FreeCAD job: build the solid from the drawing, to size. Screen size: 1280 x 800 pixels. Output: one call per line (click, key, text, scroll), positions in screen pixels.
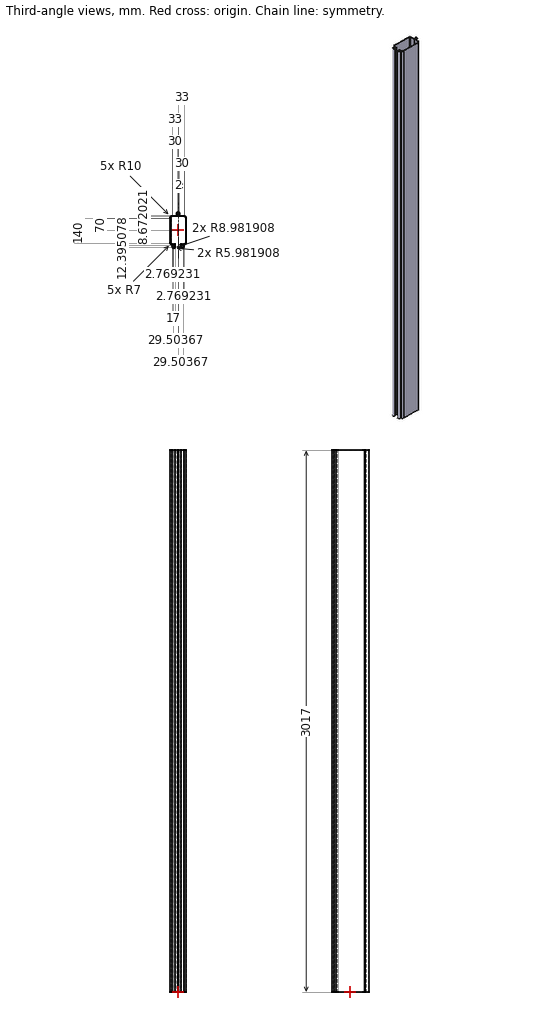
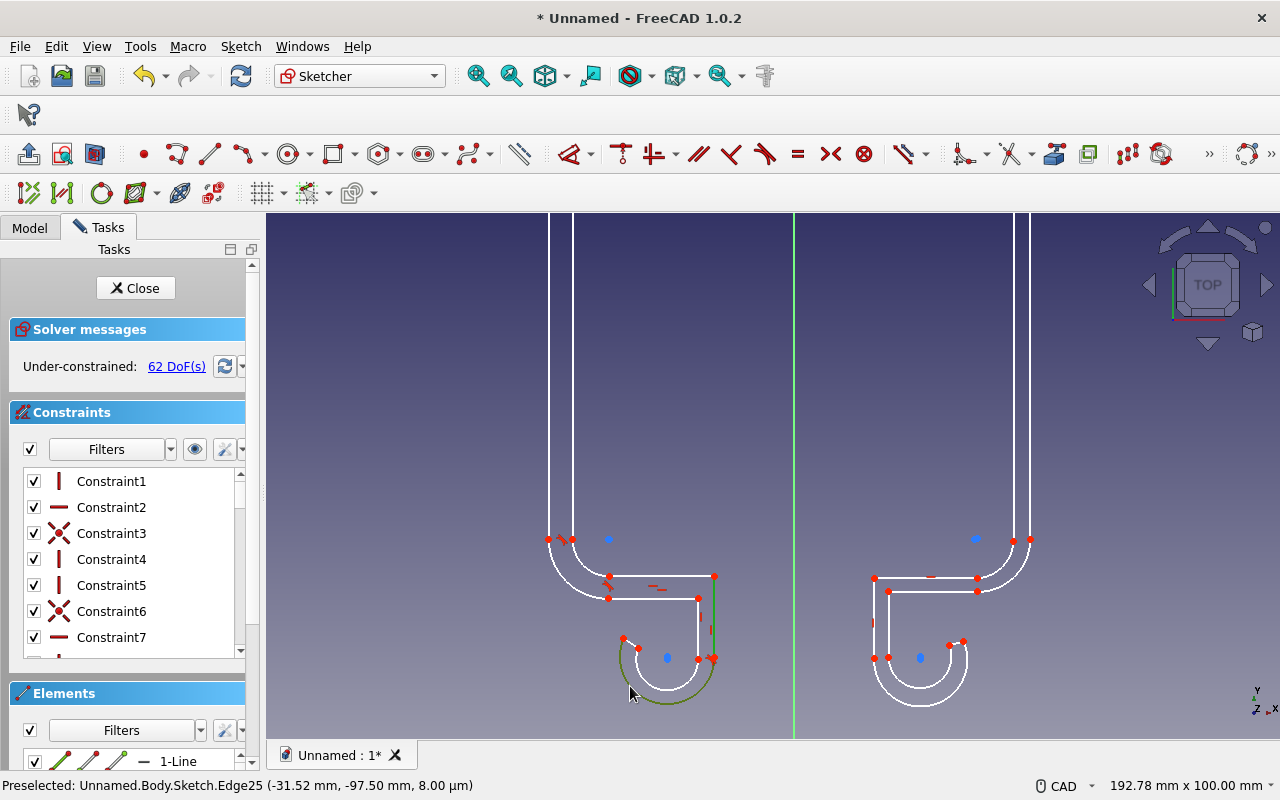
click(765, 154)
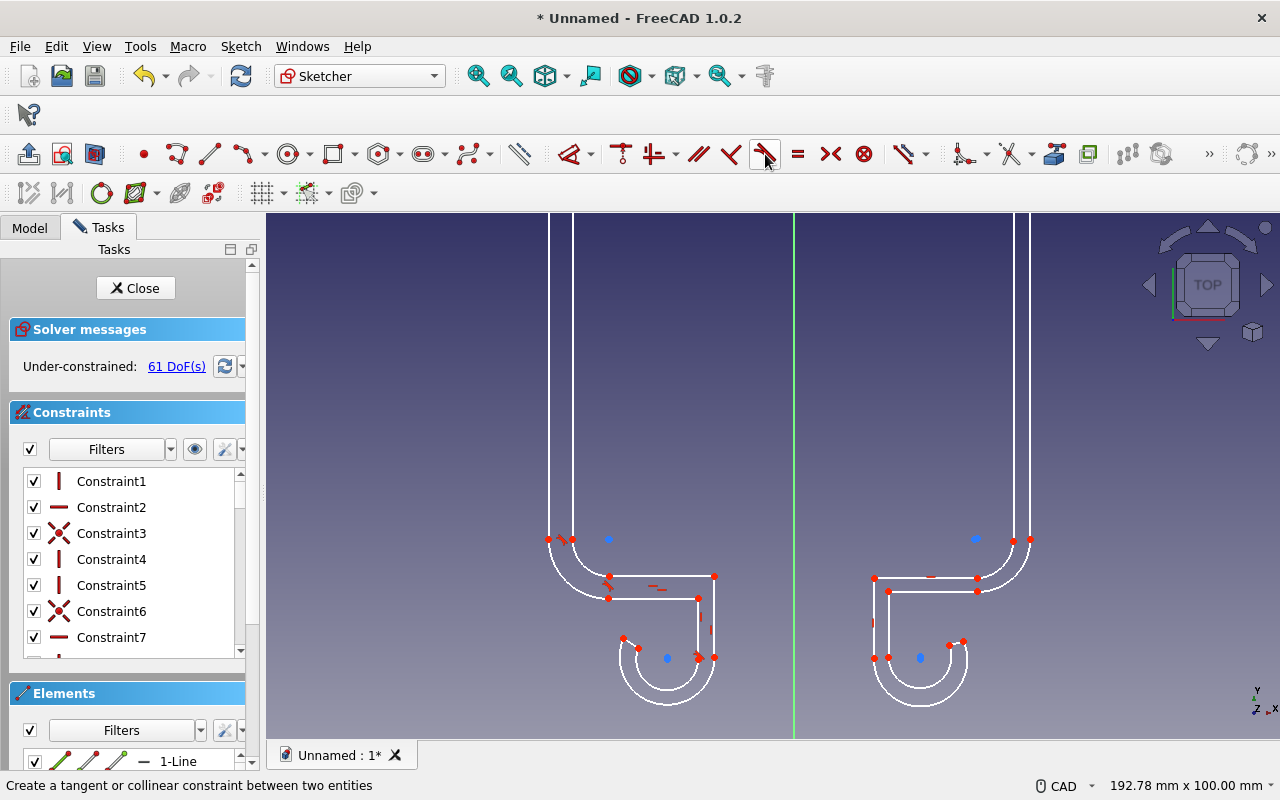
click(683, 576)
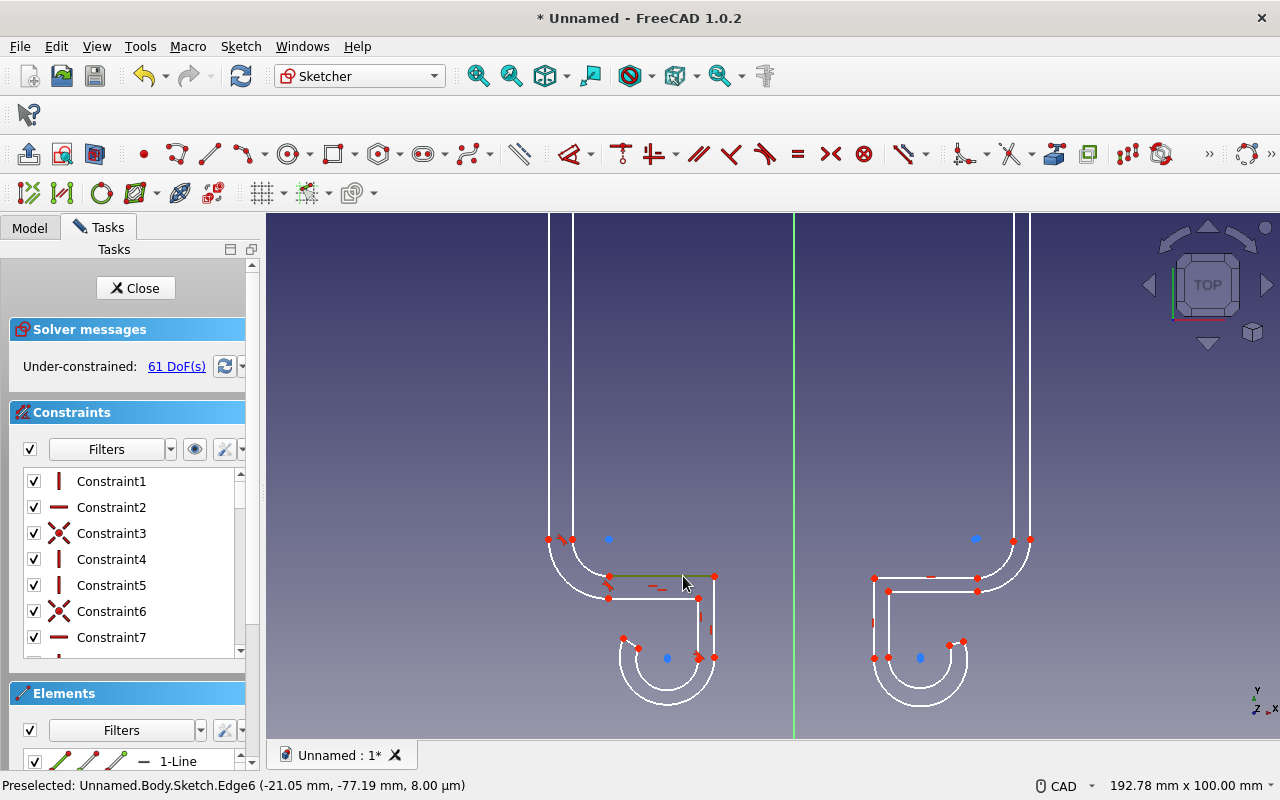
click(577, 556)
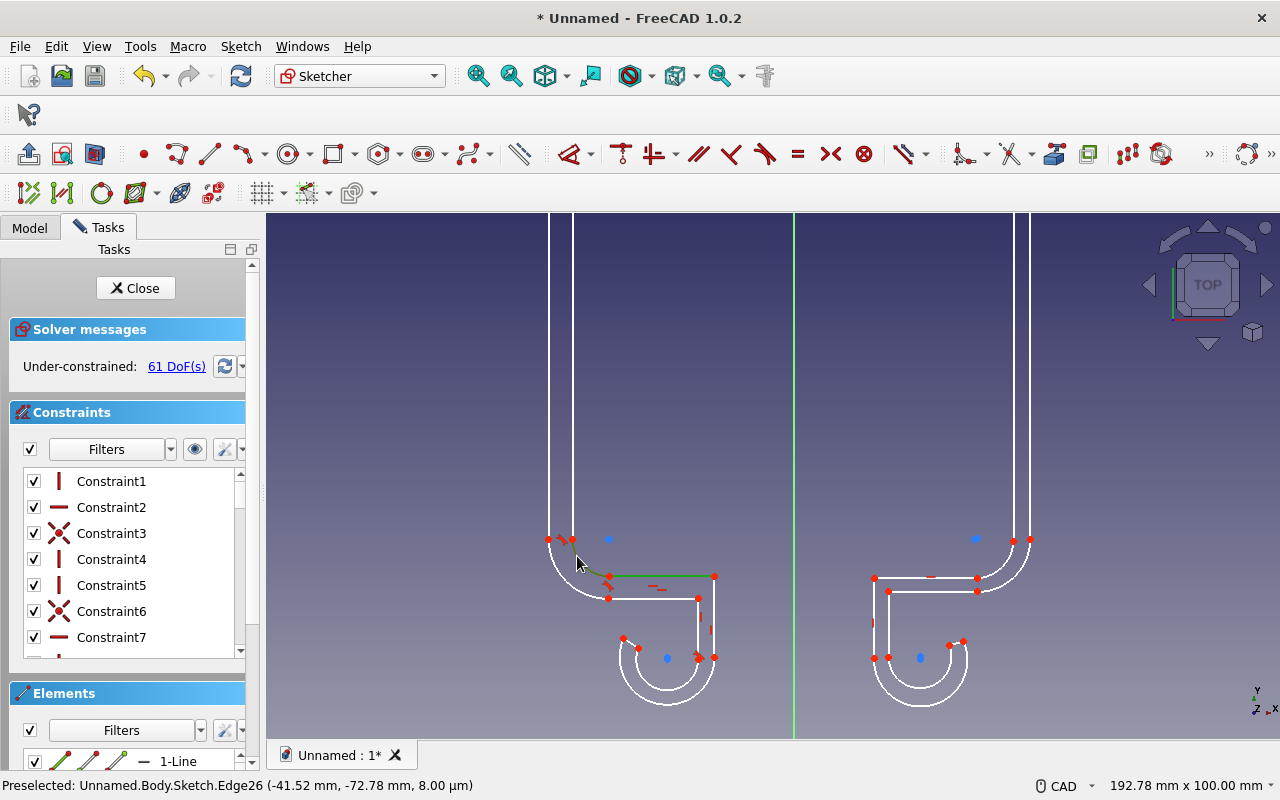
click(765, 154)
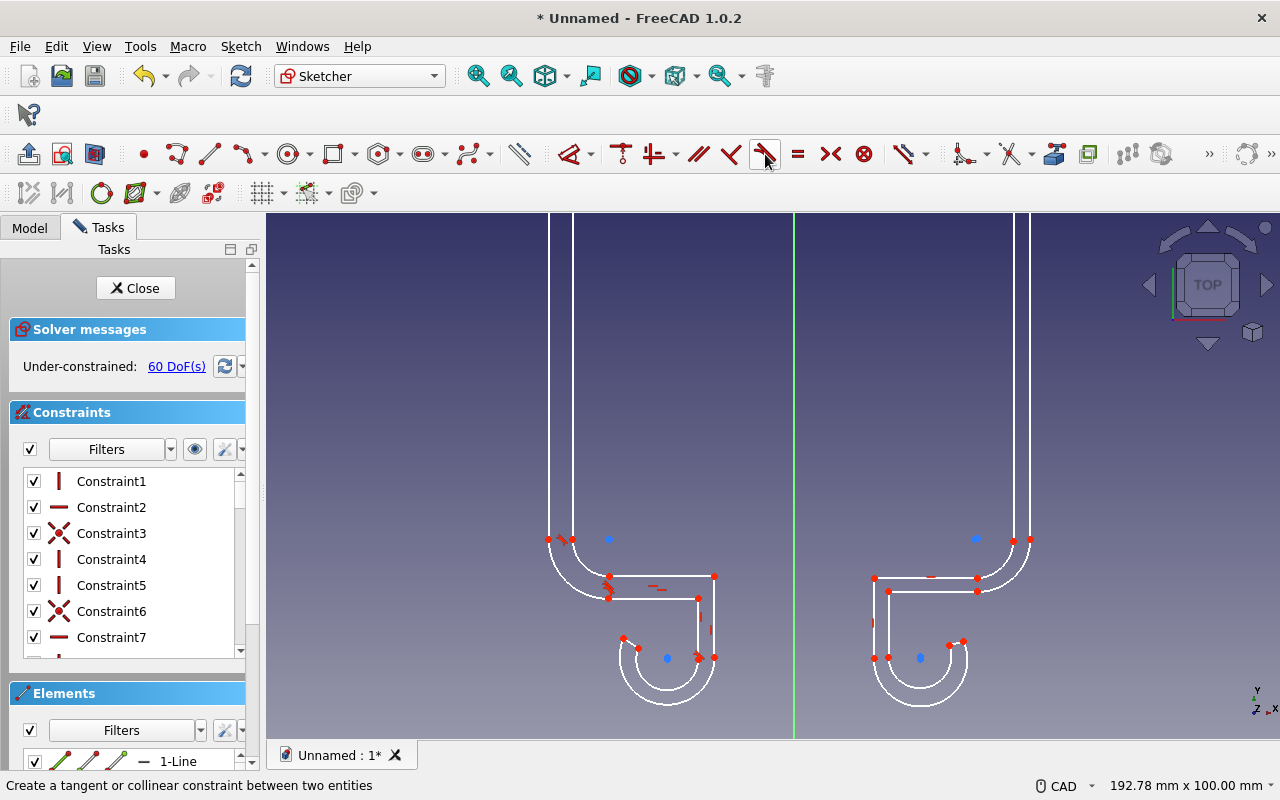
click(573, 319)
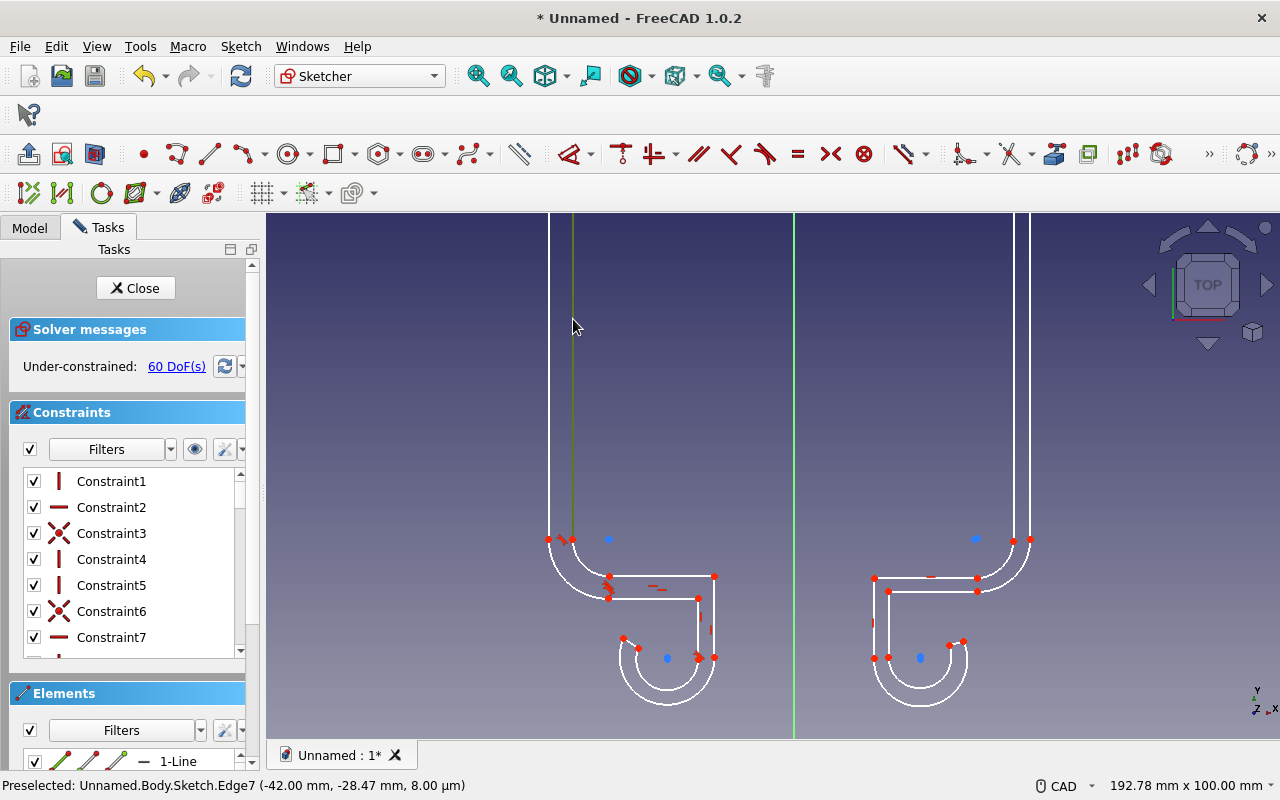
click(577, 556)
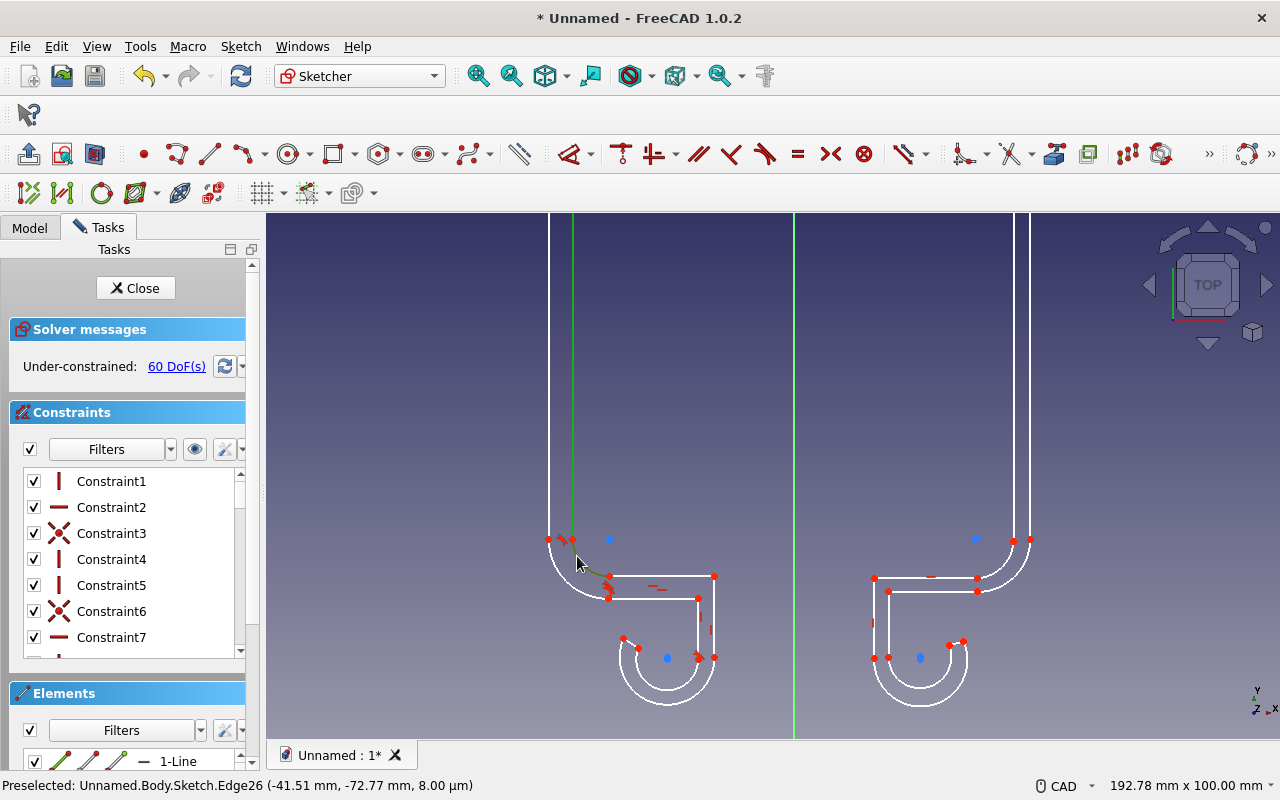
click(765, 154)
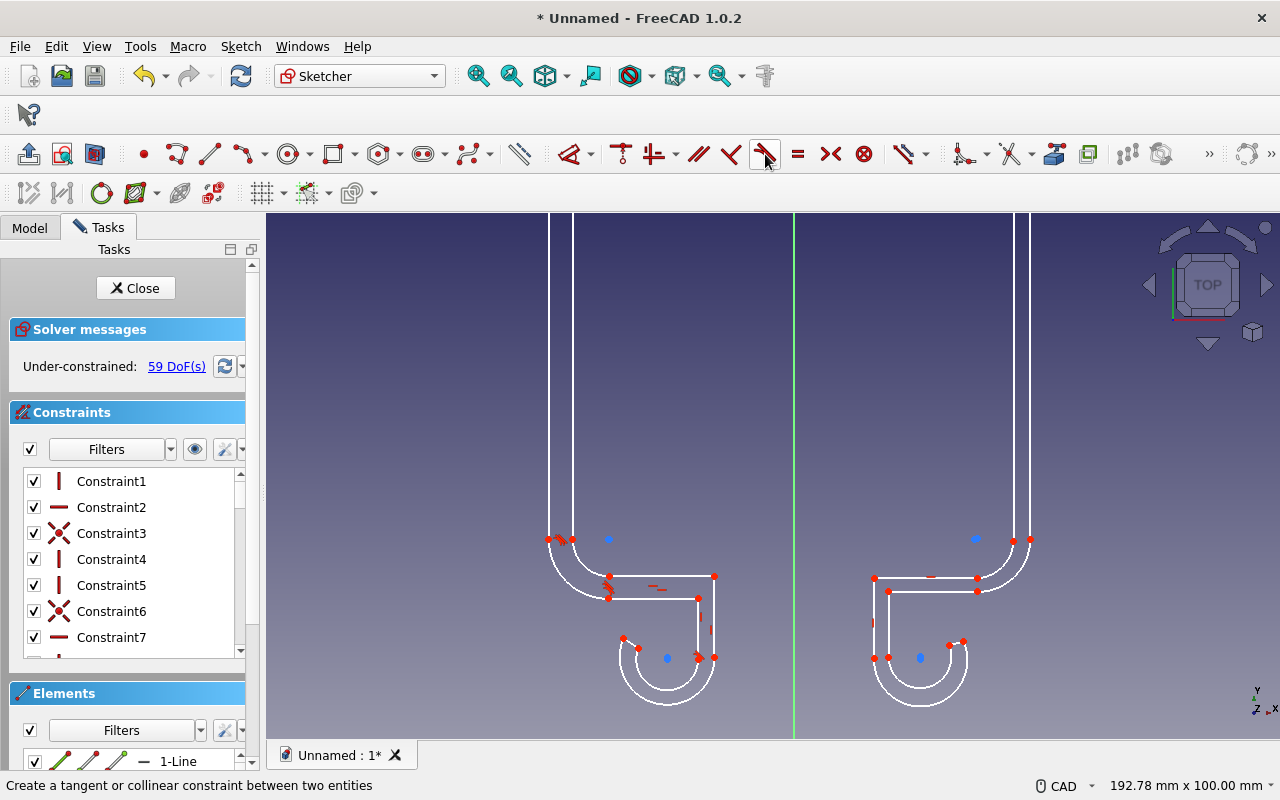
click(573, 319)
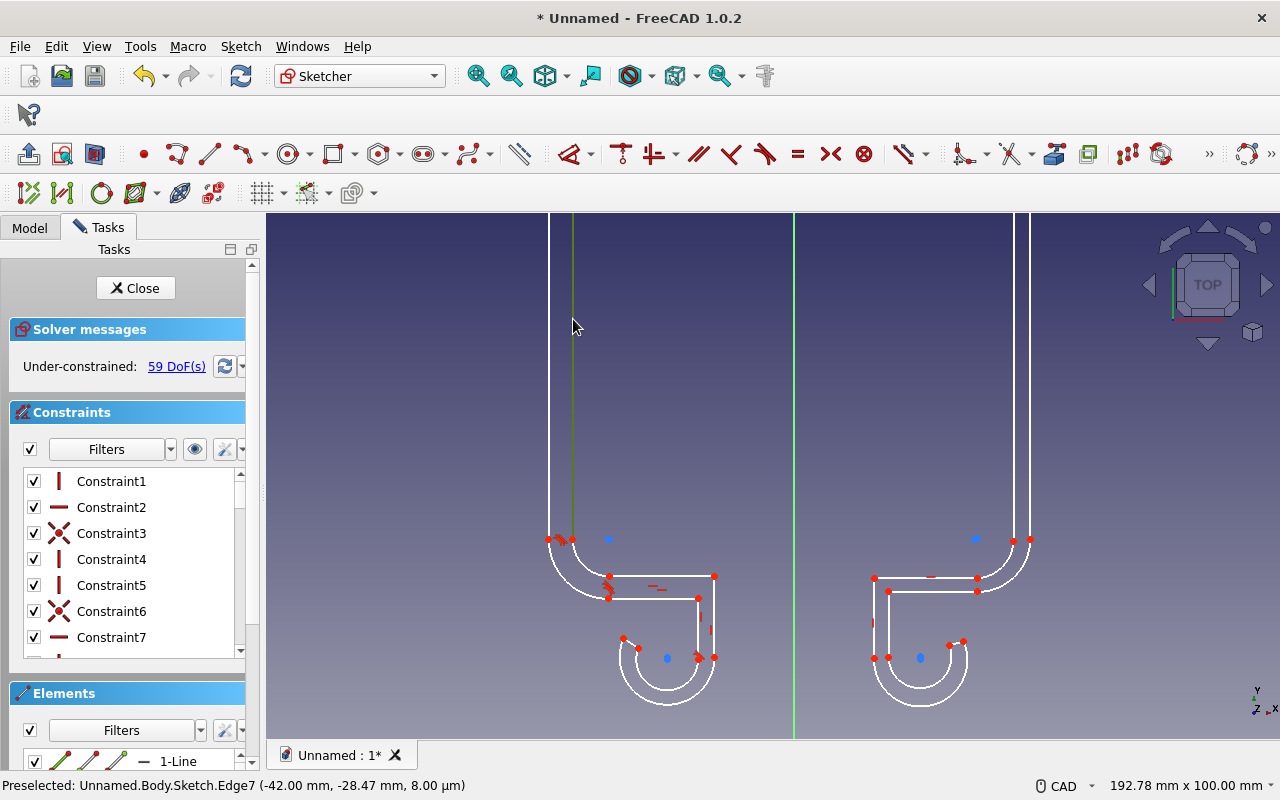
scroll(666, 609, down, 6)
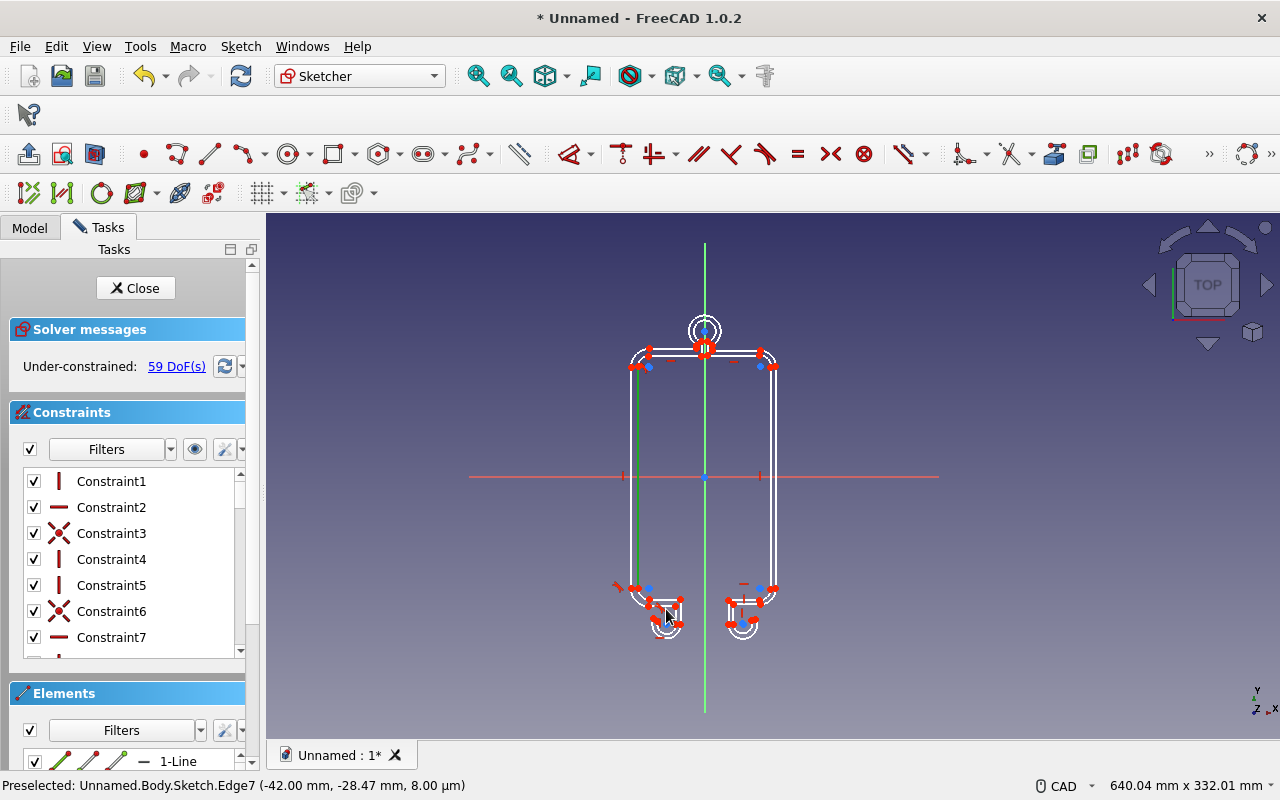
scroll(644, 357, up, 6)